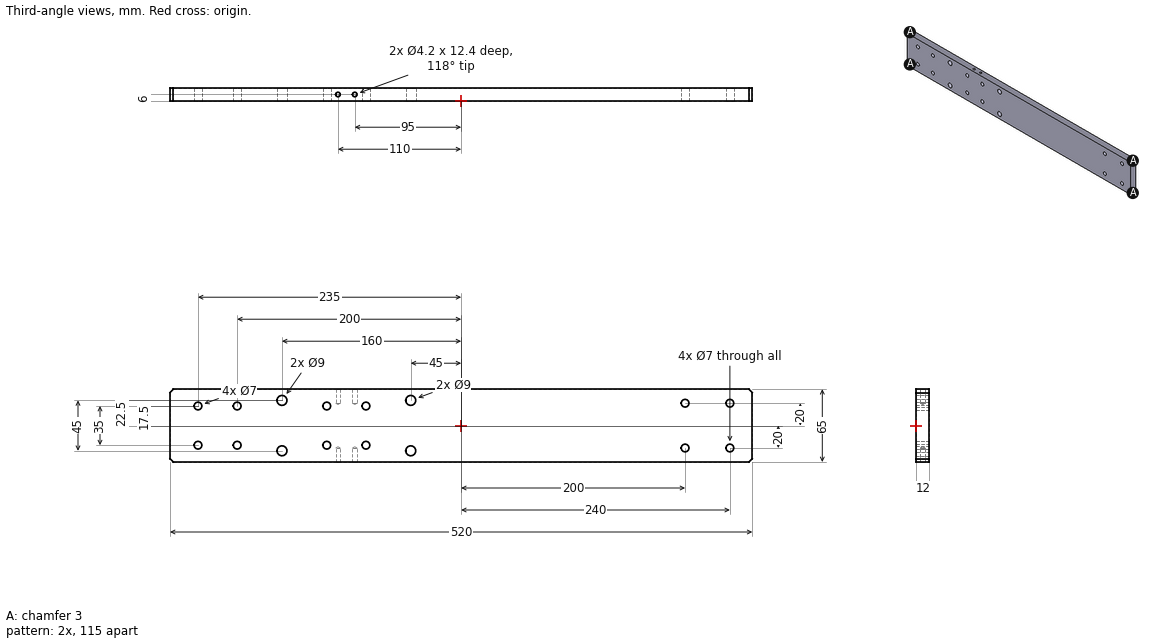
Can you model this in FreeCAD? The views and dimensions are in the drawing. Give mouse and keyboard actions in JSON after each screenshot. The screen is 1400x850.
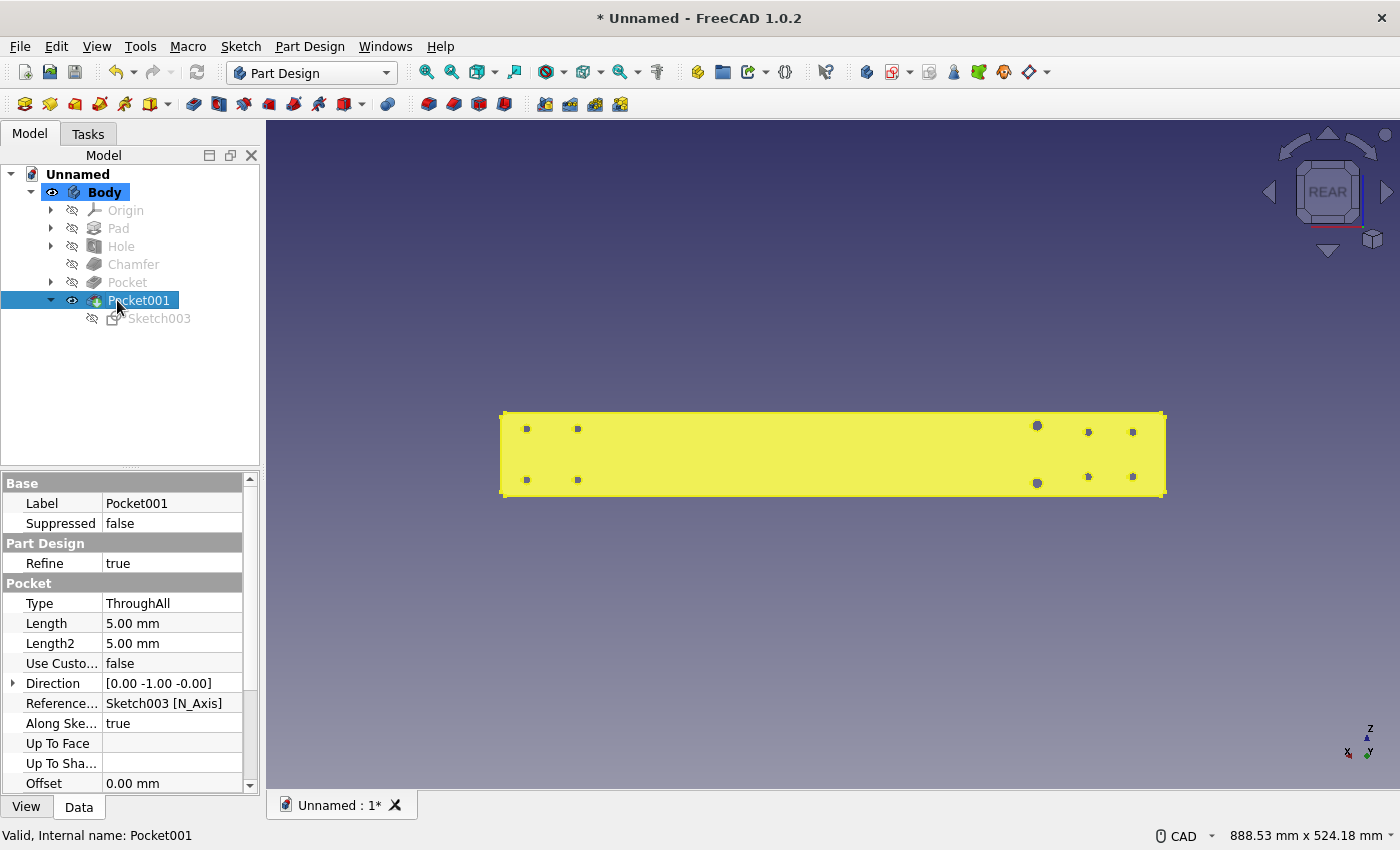
{"action": "left_click", "coordinate": [570, 104]}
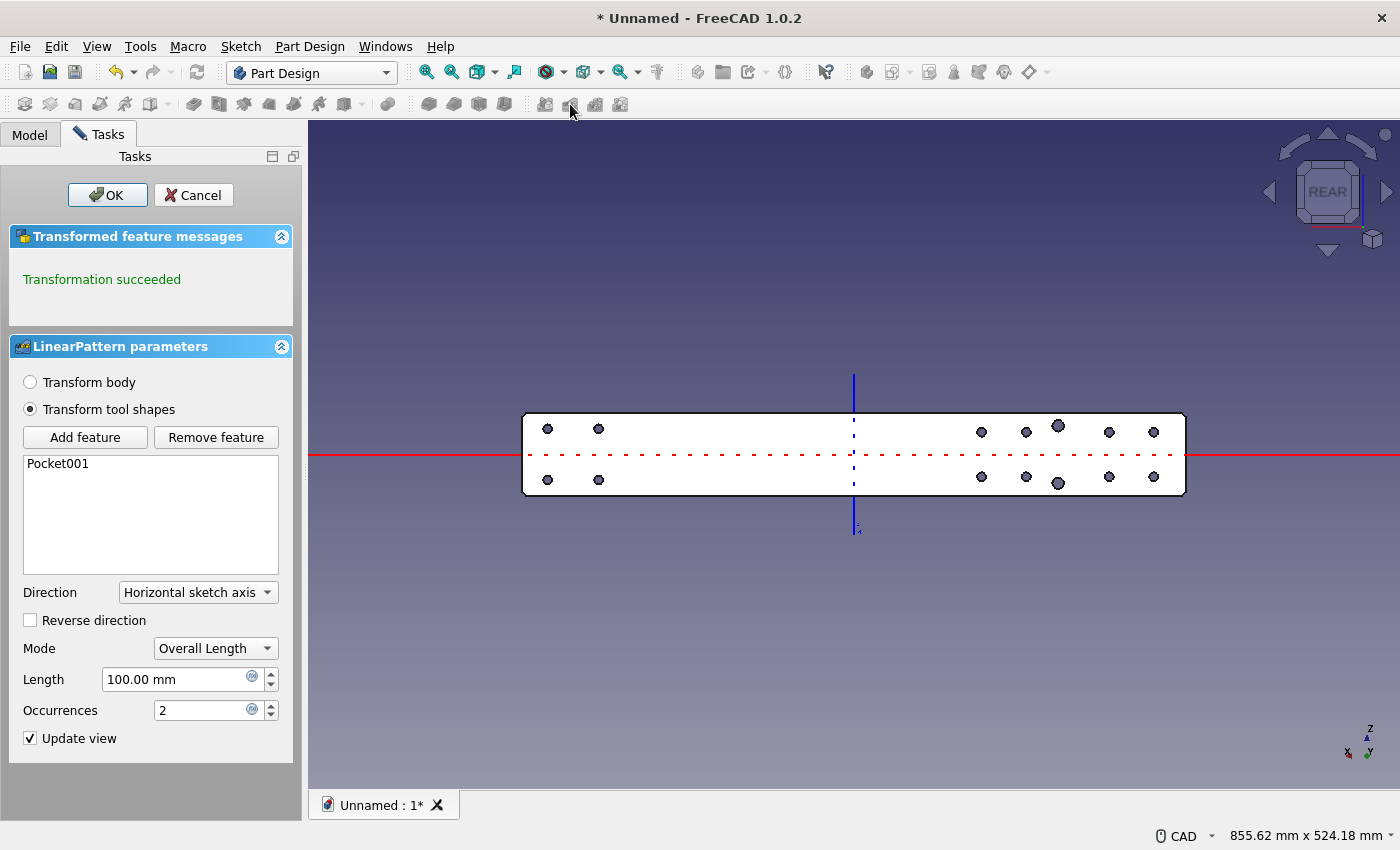
{"action": "left_click", "coordinate": [199, 592]}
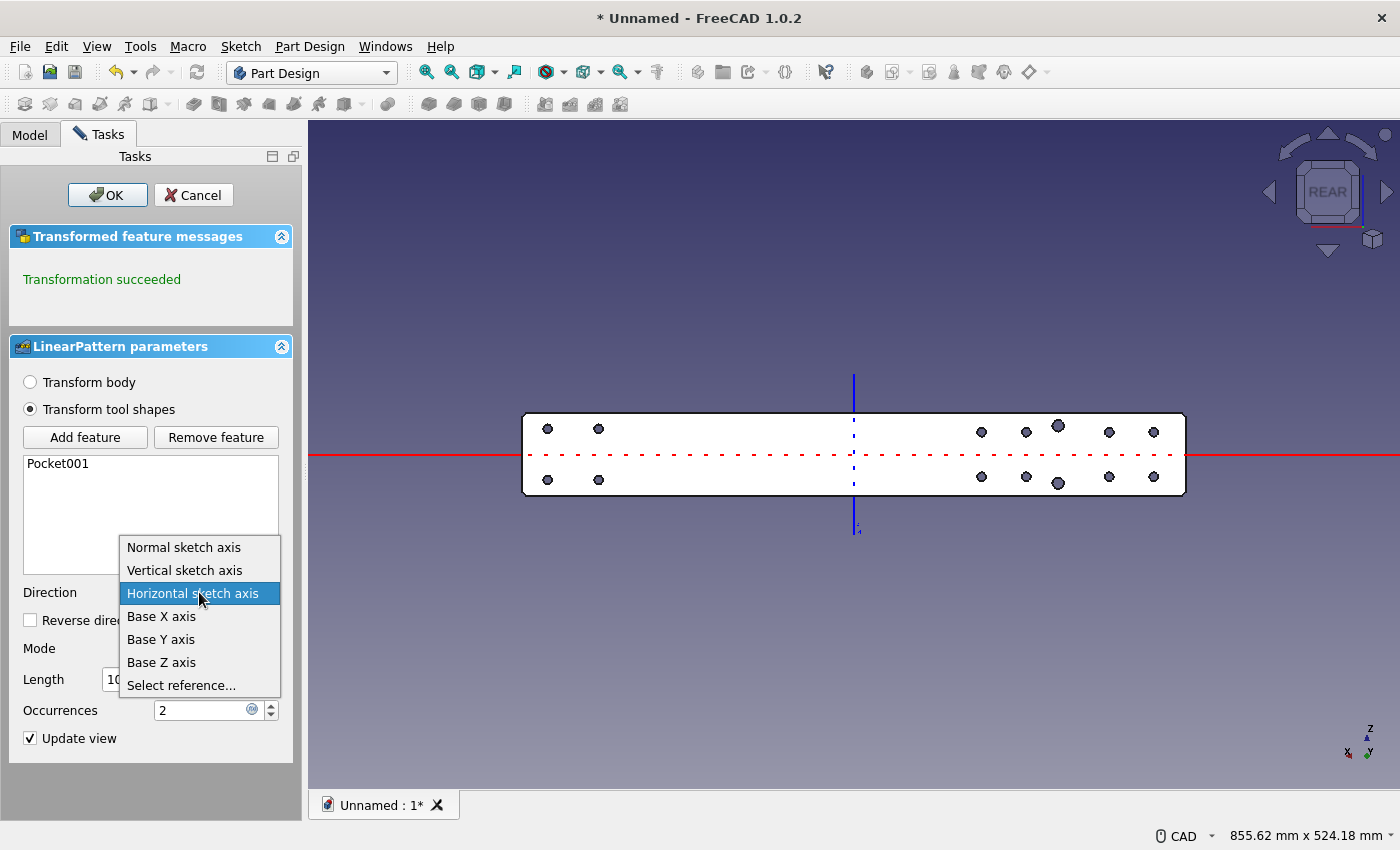
{"action": "left_click", "coordinate": [198, 616]}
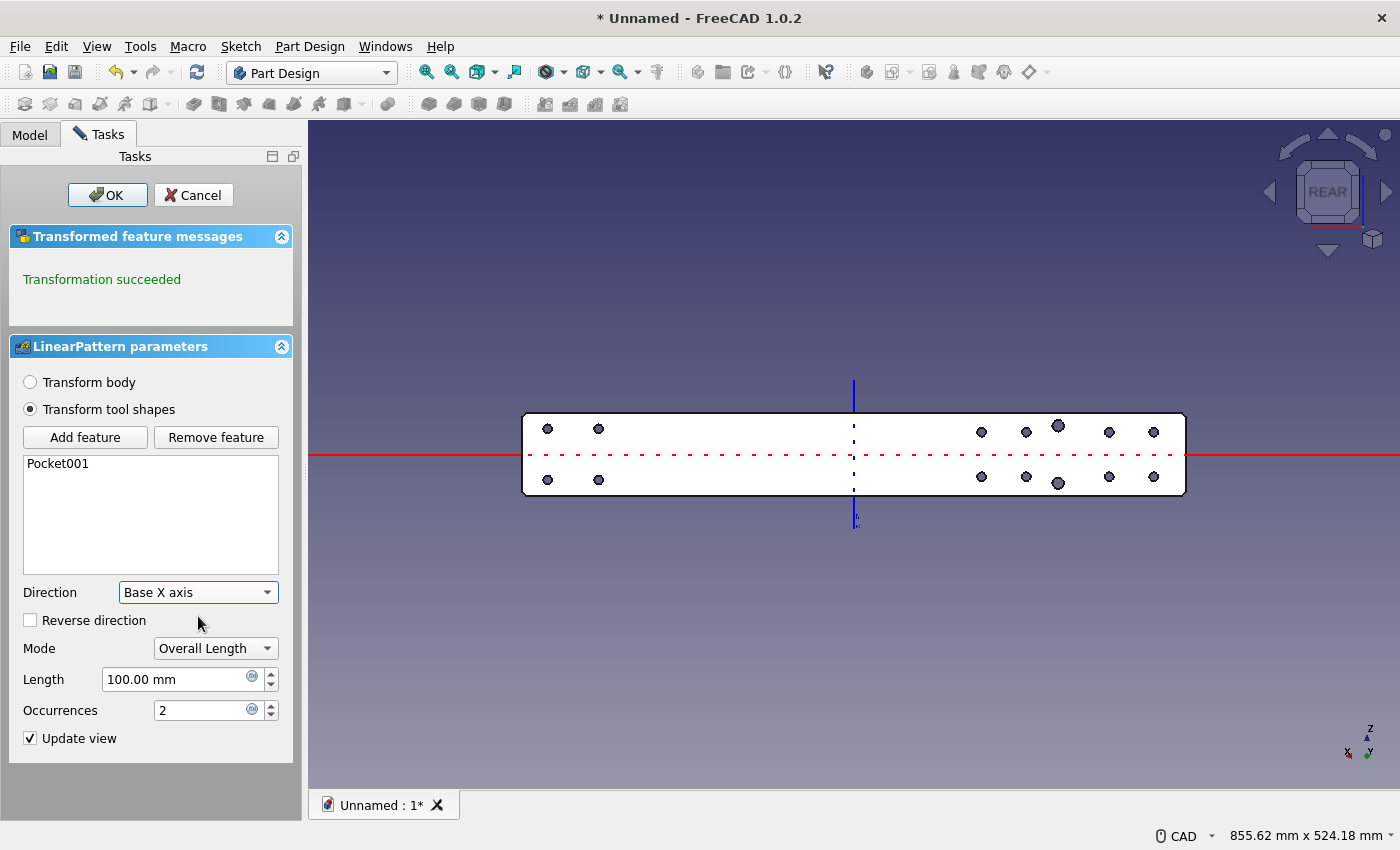
{"action": "left_click", "coordinate": [216, 648]}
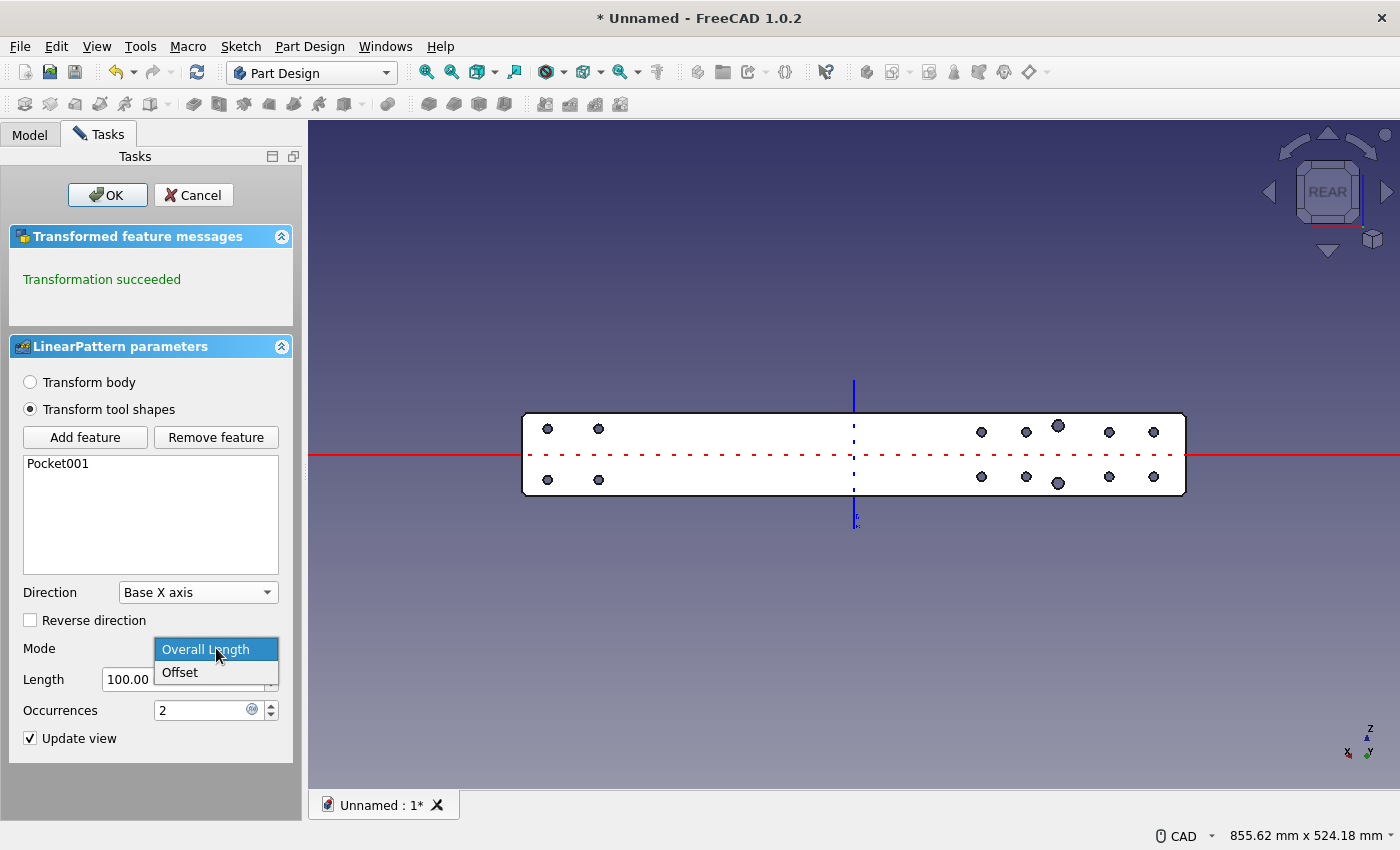
{"action": "left_click", "coordinate": [214, 672]}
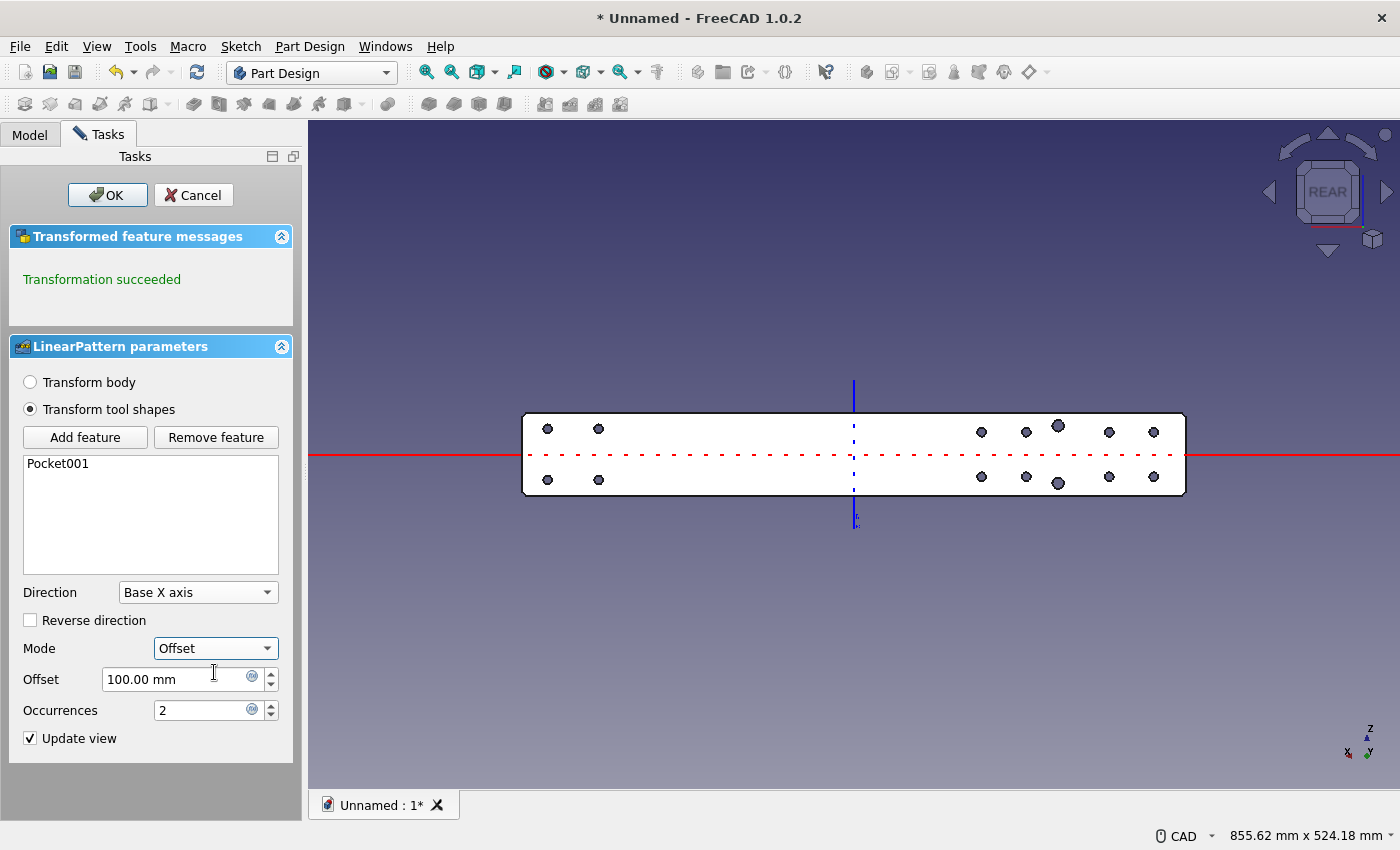
{"action": "triple_click", "coordinate": [184, 680]}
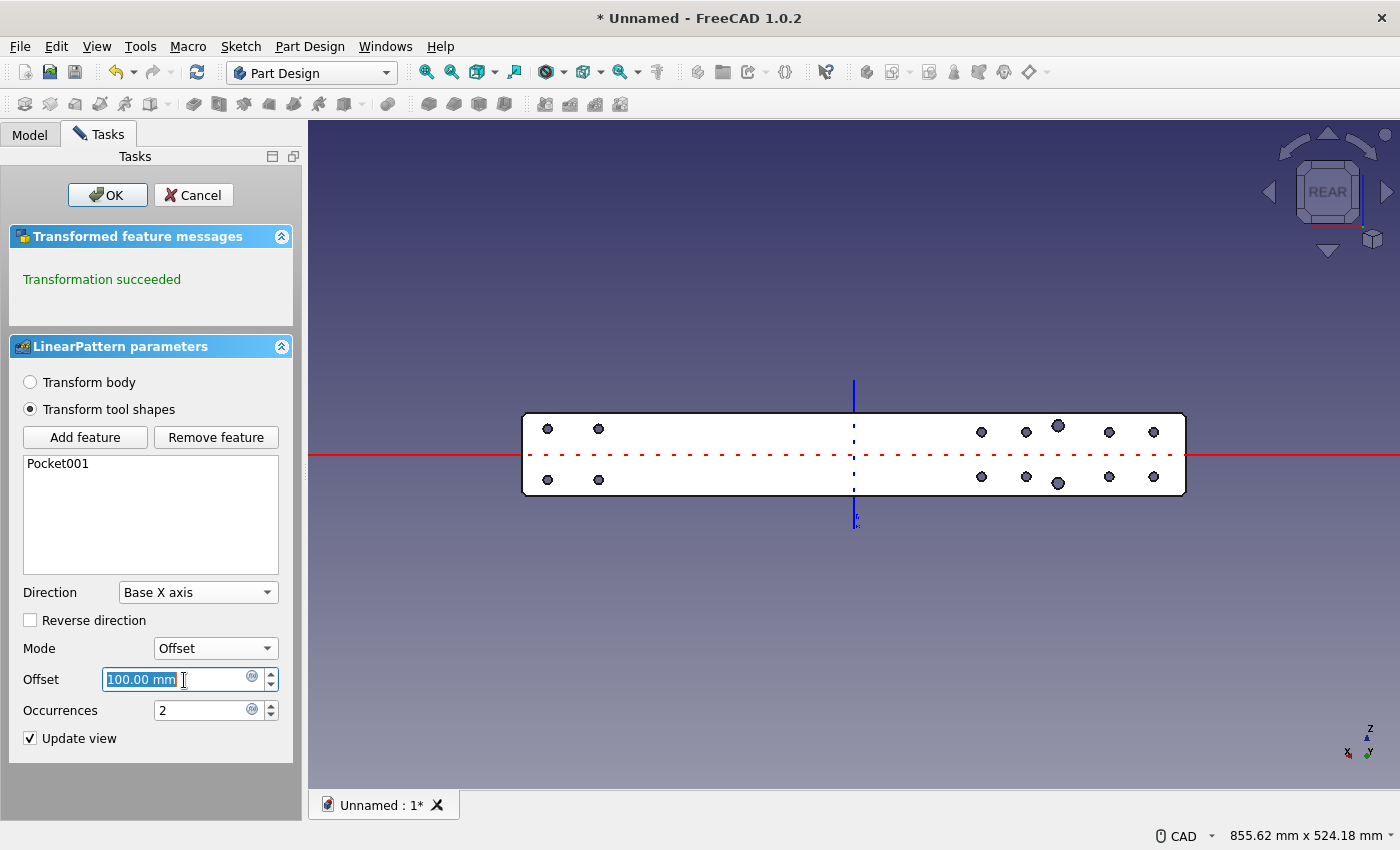
{"action": "type", "text": "115"}
{"action": "key", "text": "Tab"}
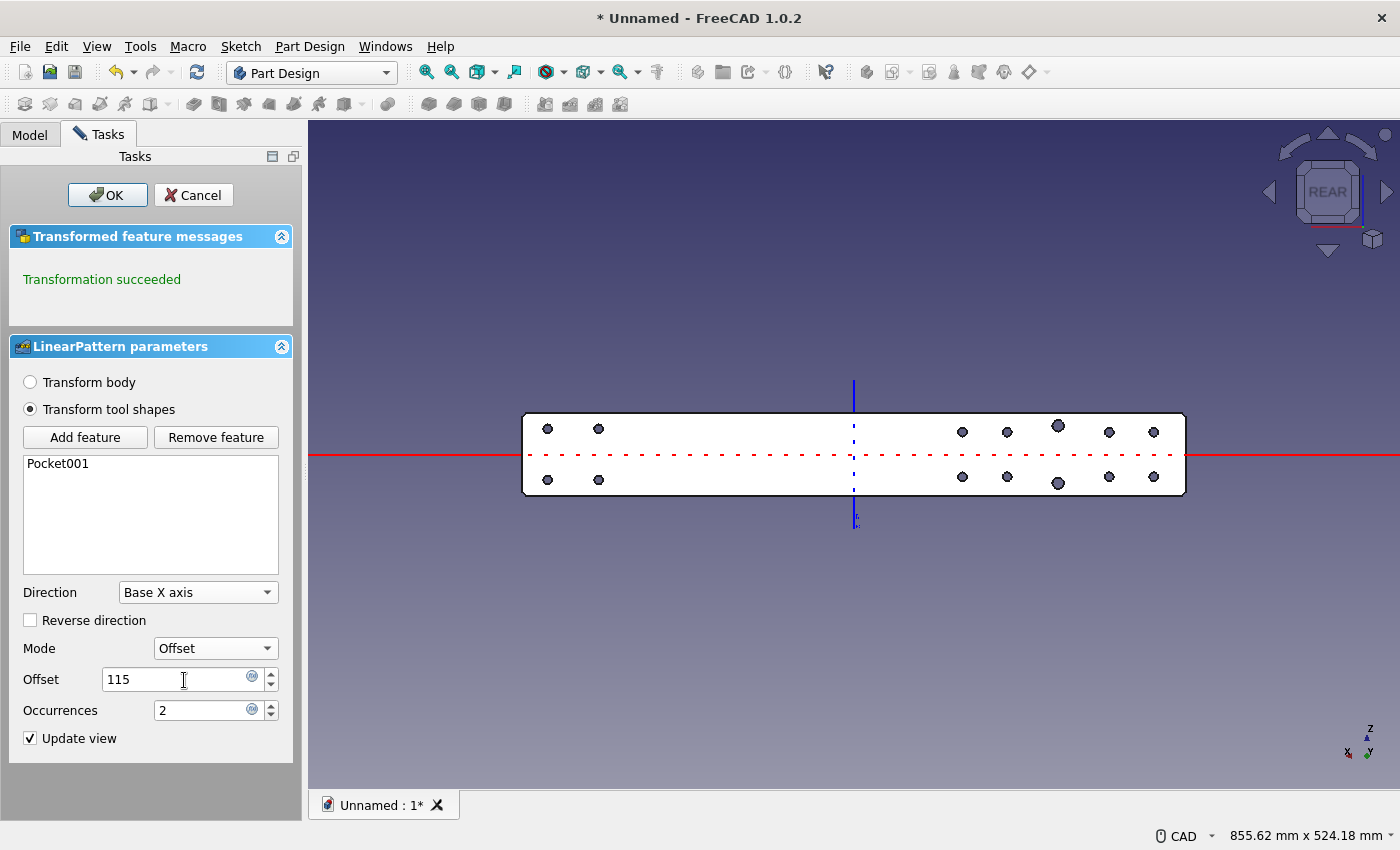
{"action": "triple_click", "coordinate": [210, 710]}